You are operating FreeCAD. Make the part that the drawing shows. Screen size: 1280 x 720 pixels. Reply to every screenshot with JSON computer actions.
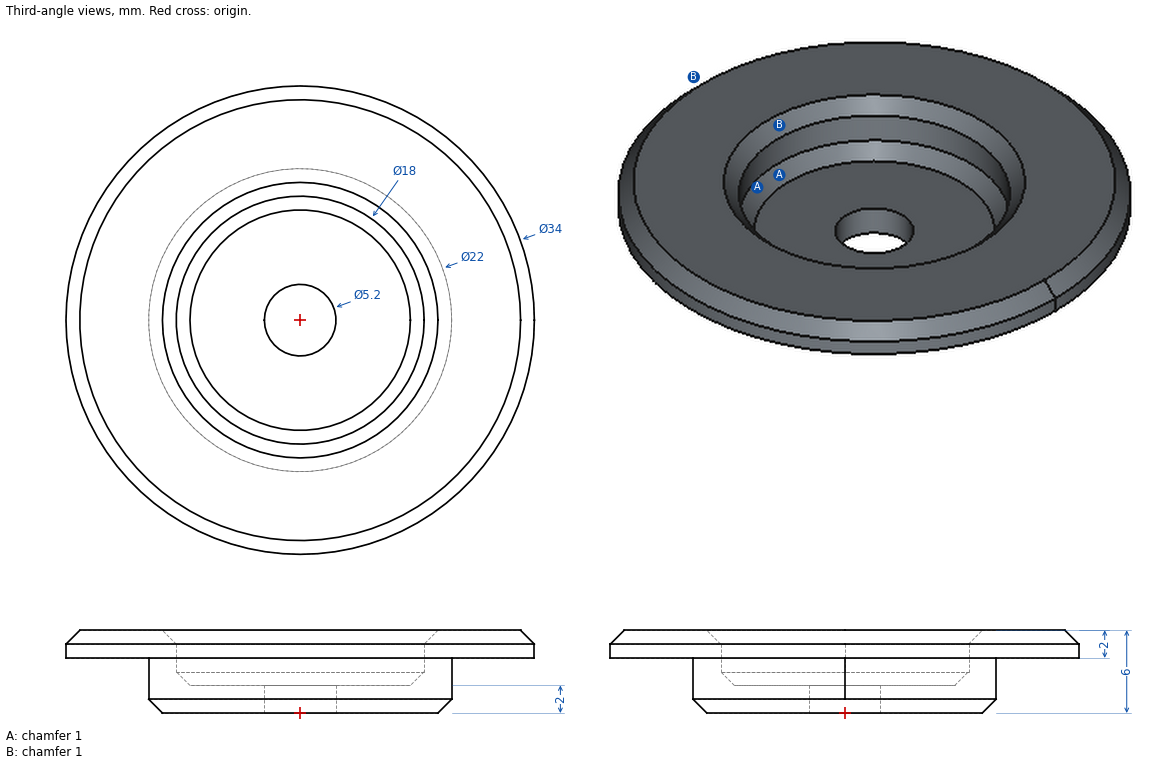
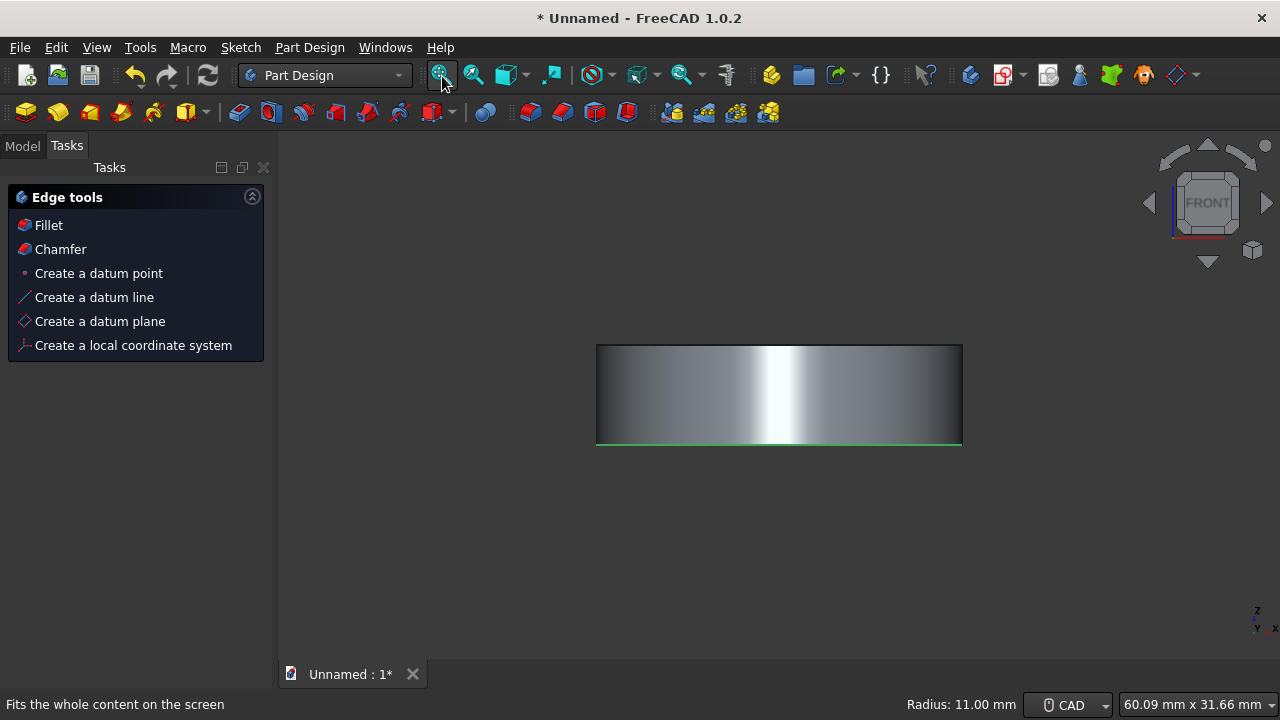
{"action": "key", "text": "3"}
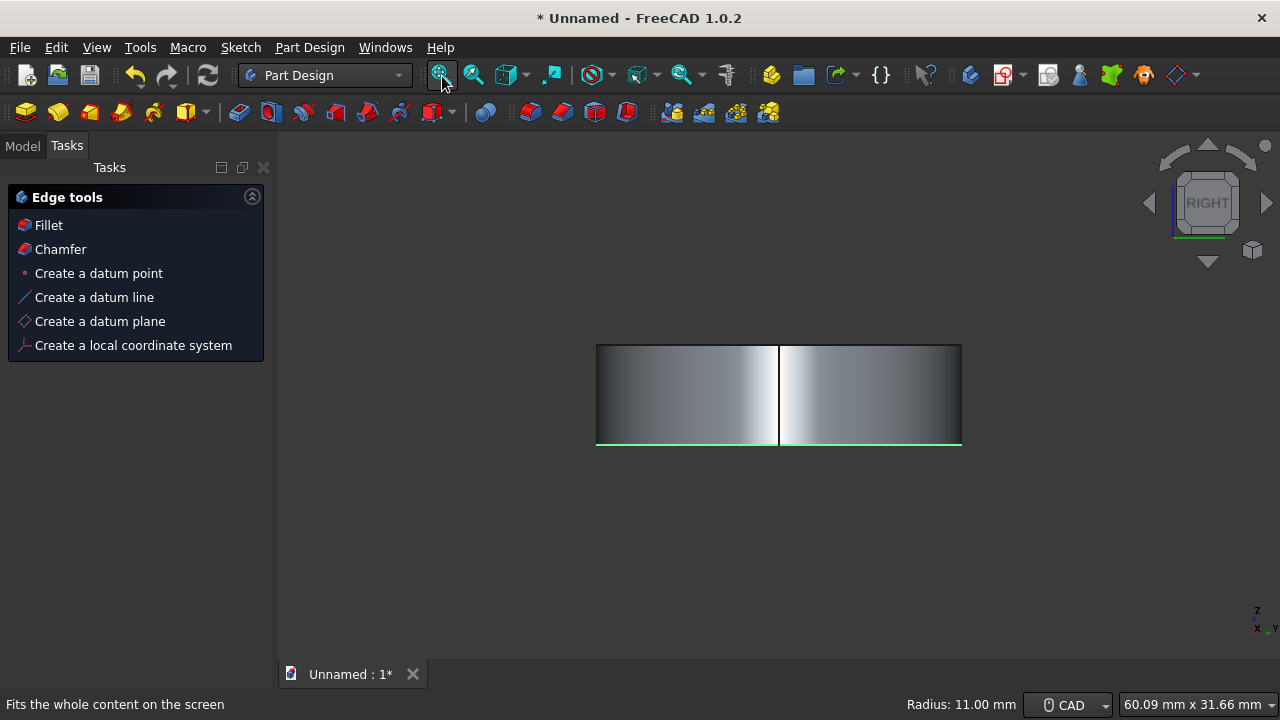
{"action": "left_click", "coordinate": [442, 76]}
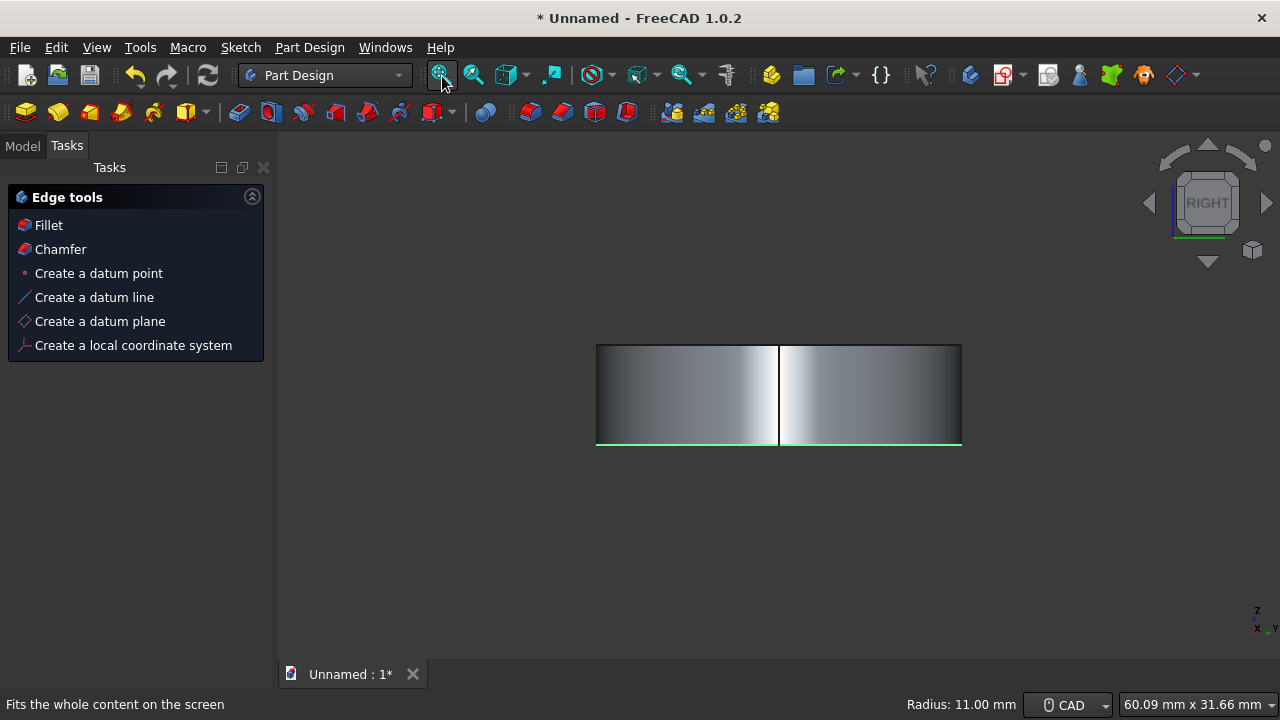
{"action": "key", "text": "5"}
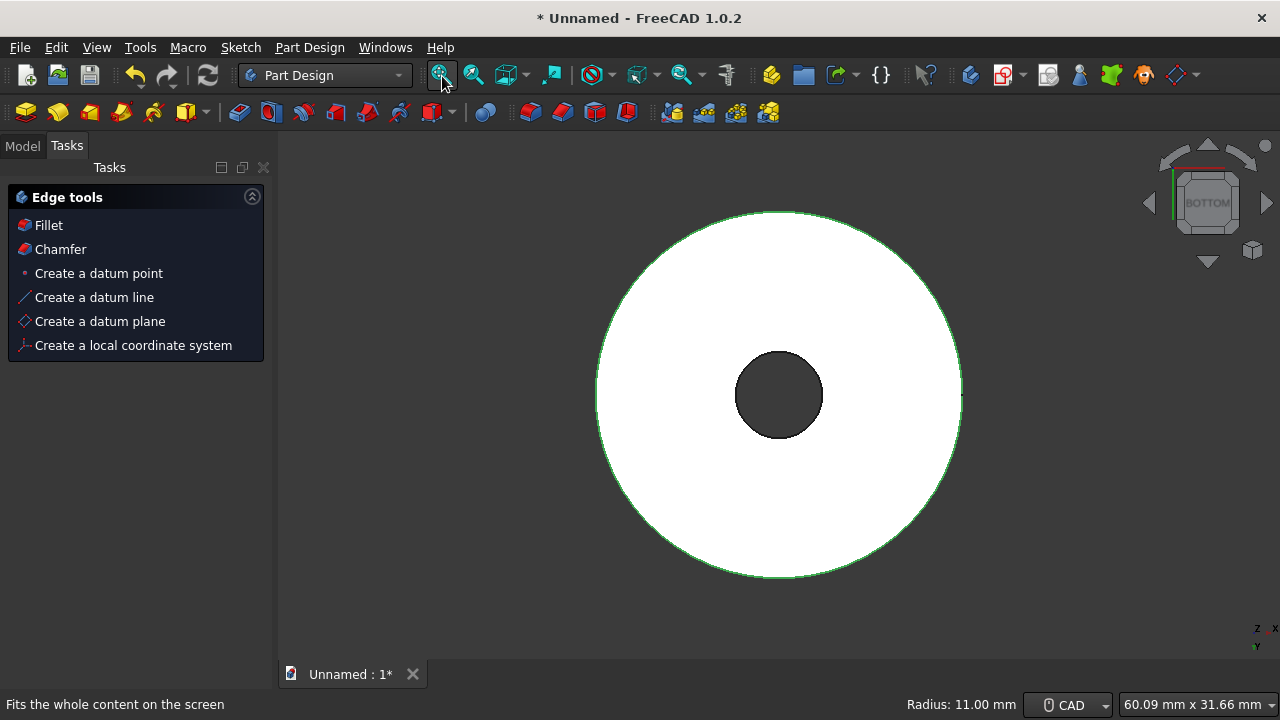
{"action": "key", "text": "4"}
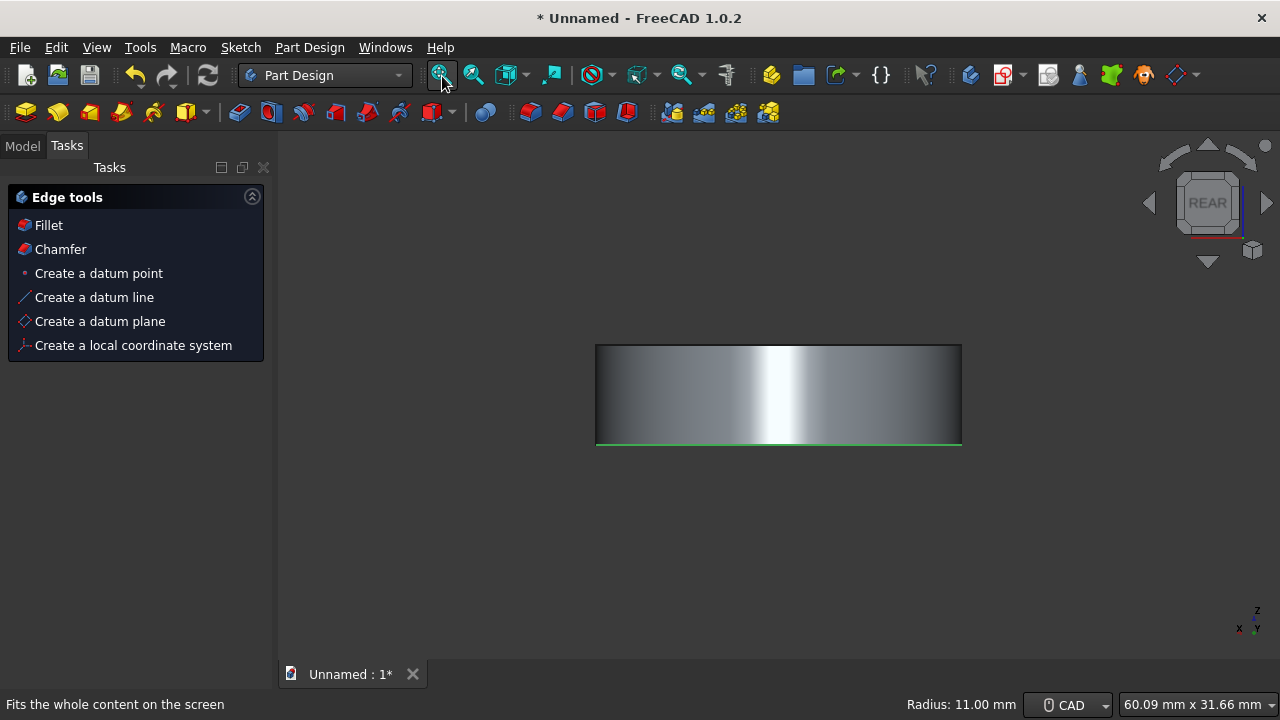
{"action": "left_click", "coordinate": [442, 76]}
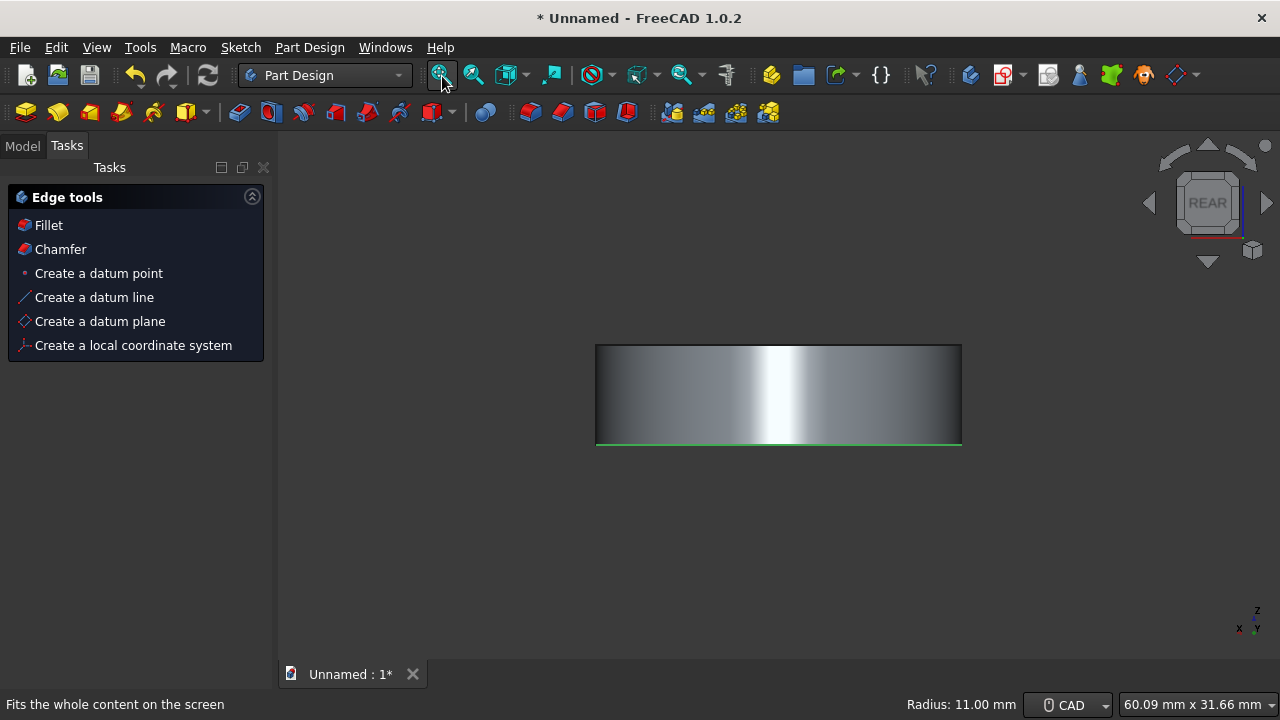
{"action": "key", "text": "6"}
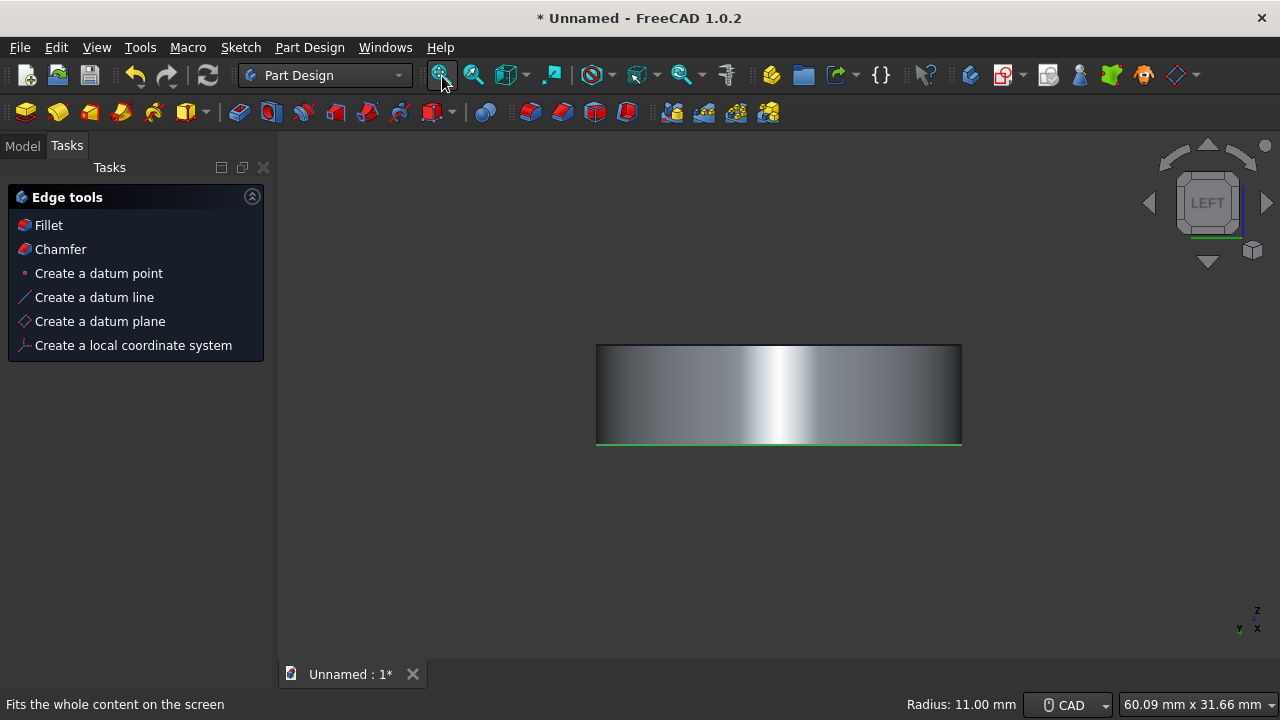
{"action": "left_click", "coordinate": [442, 76]}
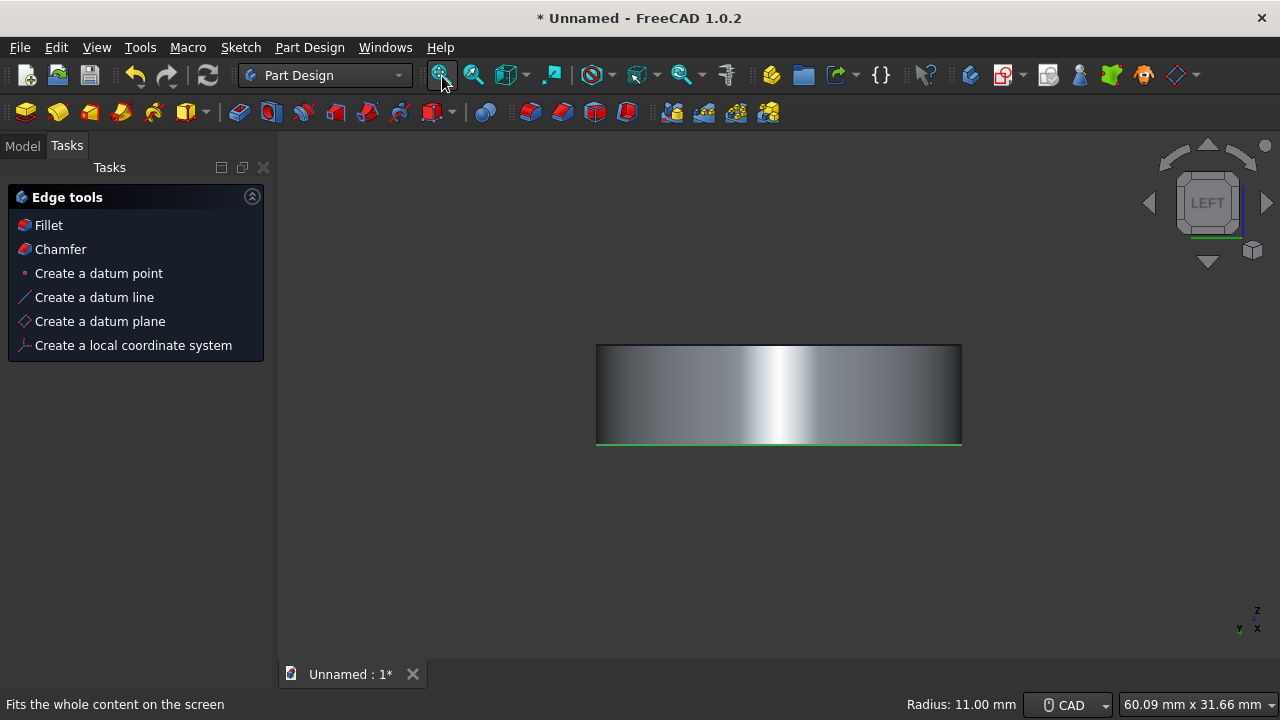
{"action": "key", "text": "v 3"}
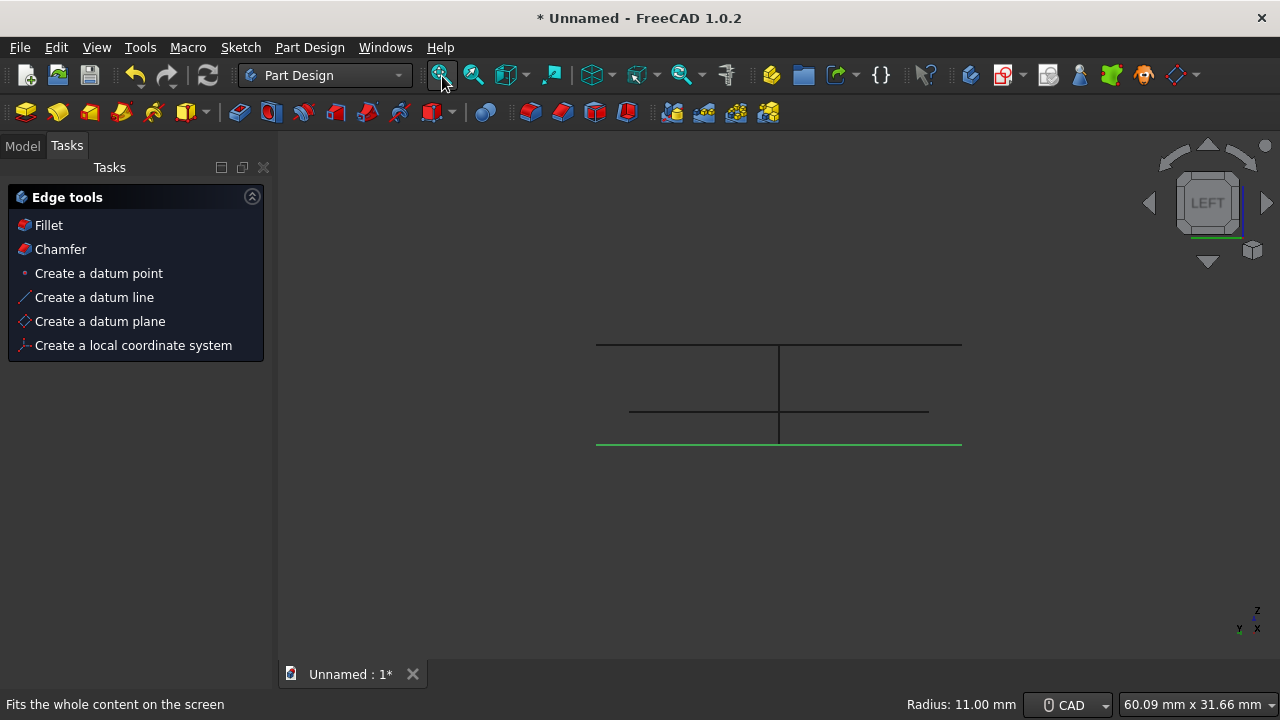
{"action": "key", "text": "0"}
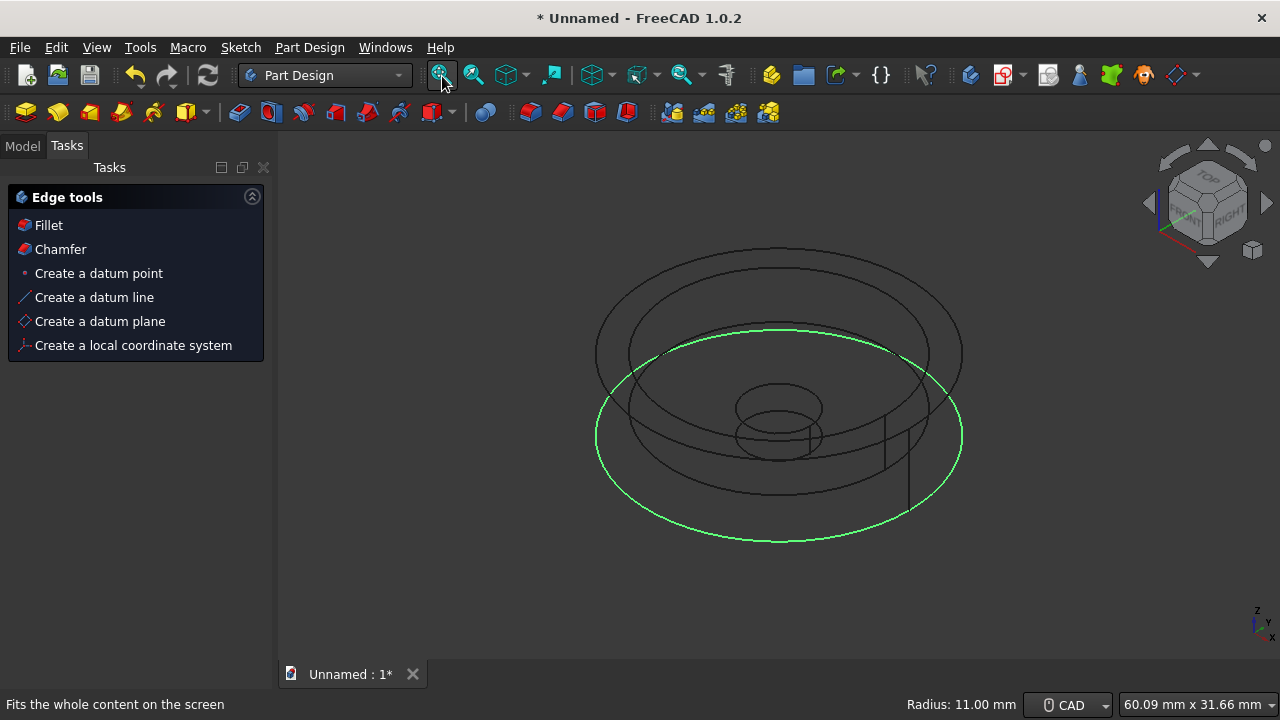
{"action": "left_click", "coordinate": [673, 346], "text": "ctrl"}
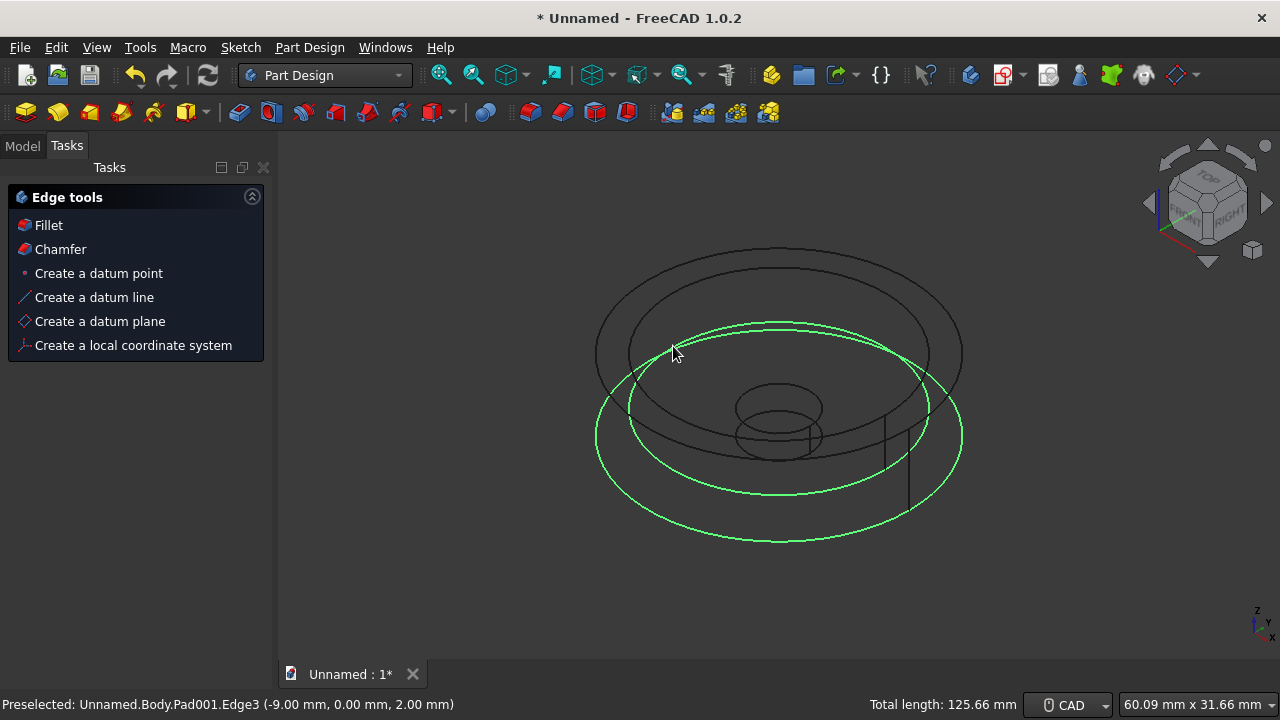
{"action": "key", "text": "v 1"}